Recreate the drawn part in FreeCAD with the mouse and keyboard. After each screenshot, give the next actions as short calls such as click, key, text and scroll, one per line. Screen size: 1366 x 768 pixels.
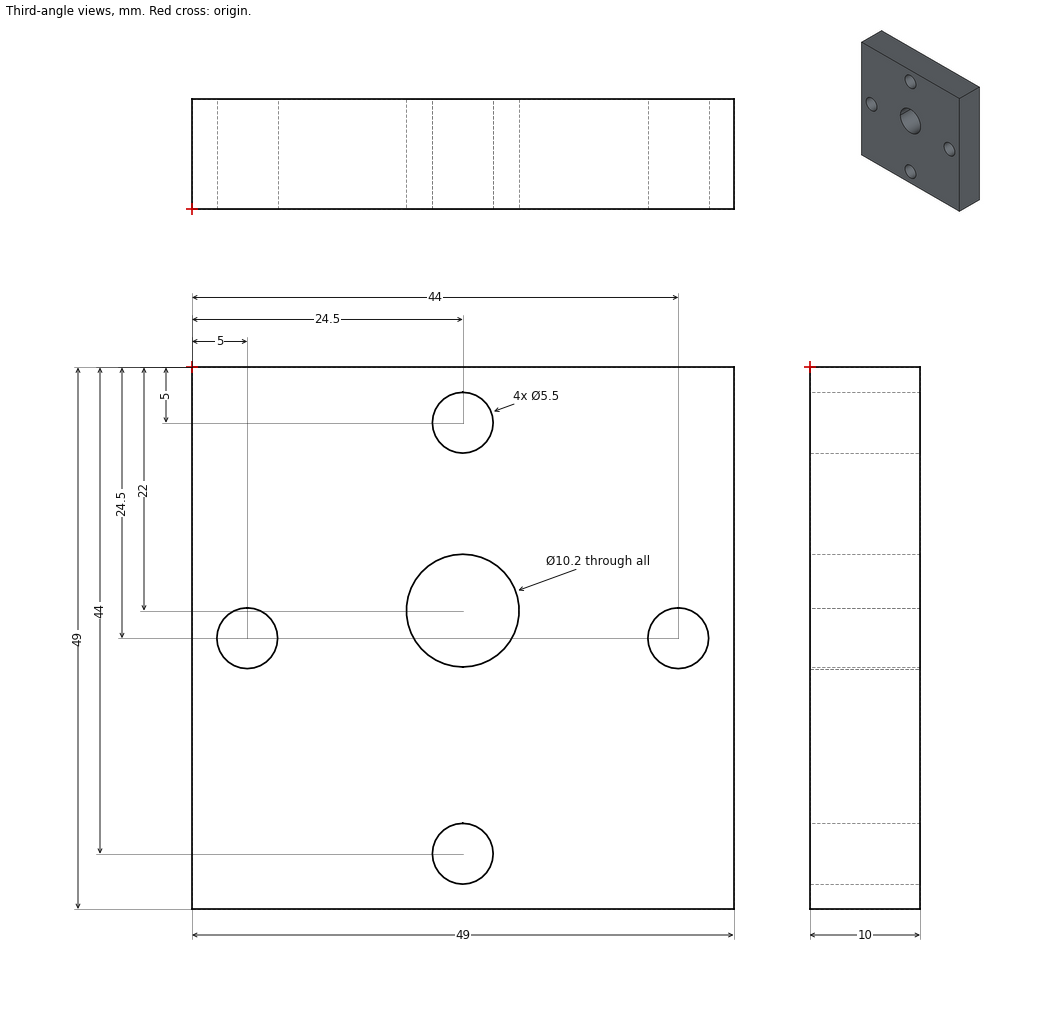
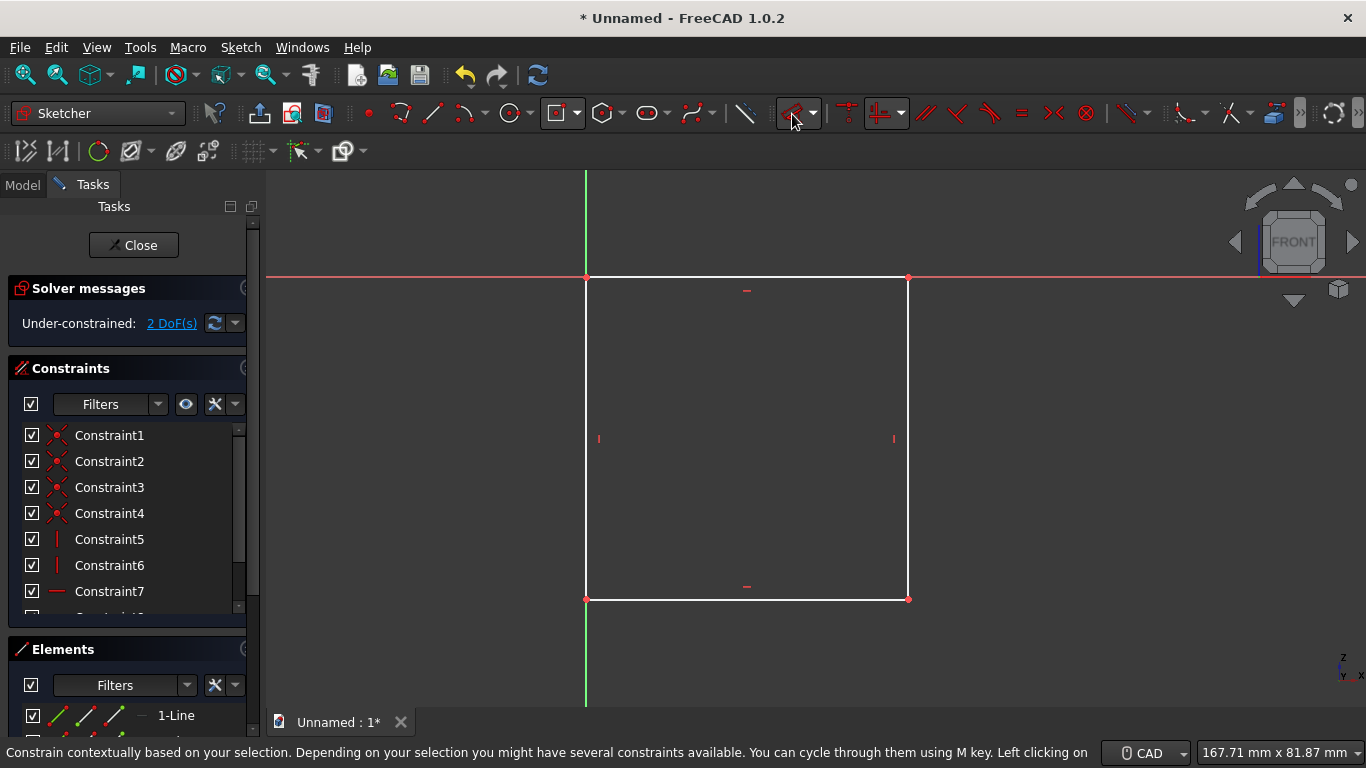
click(586, 374)
click(552, 439)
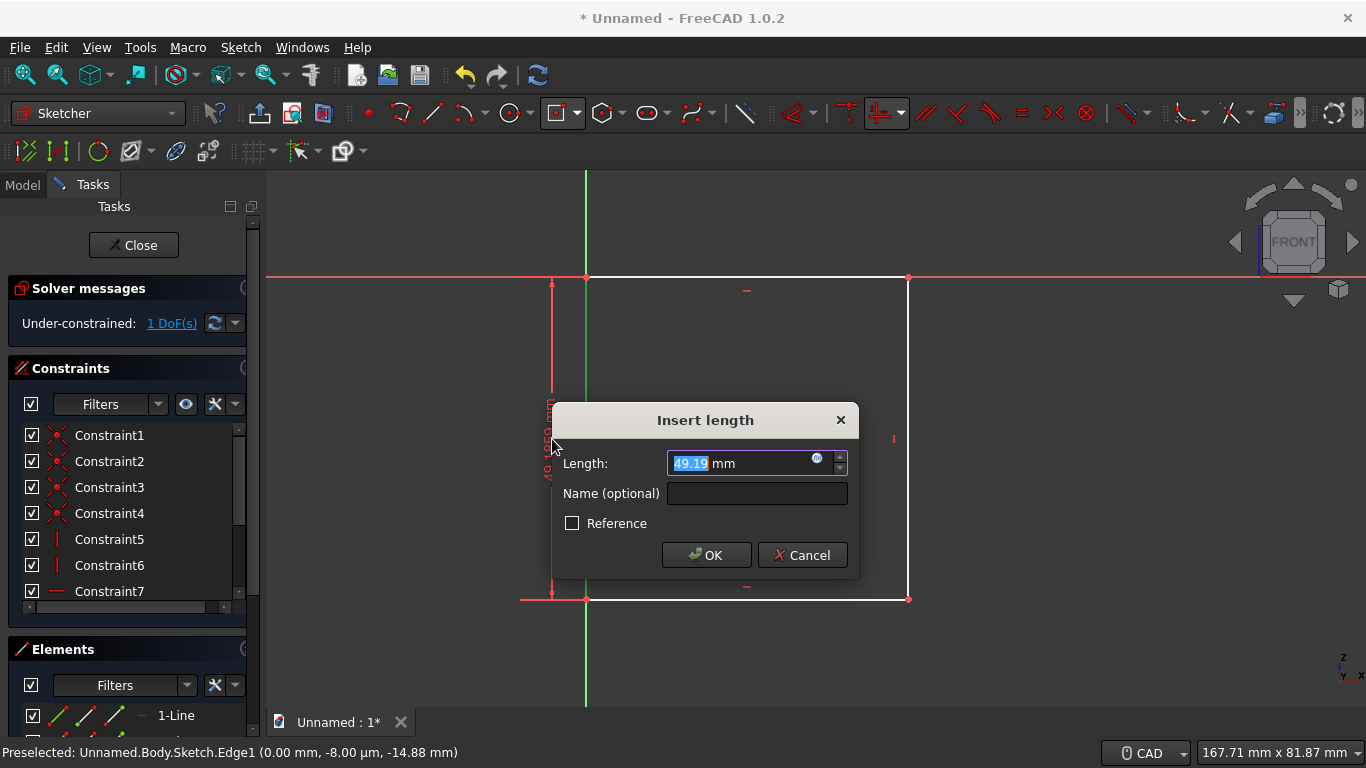
text(49)
key(Return)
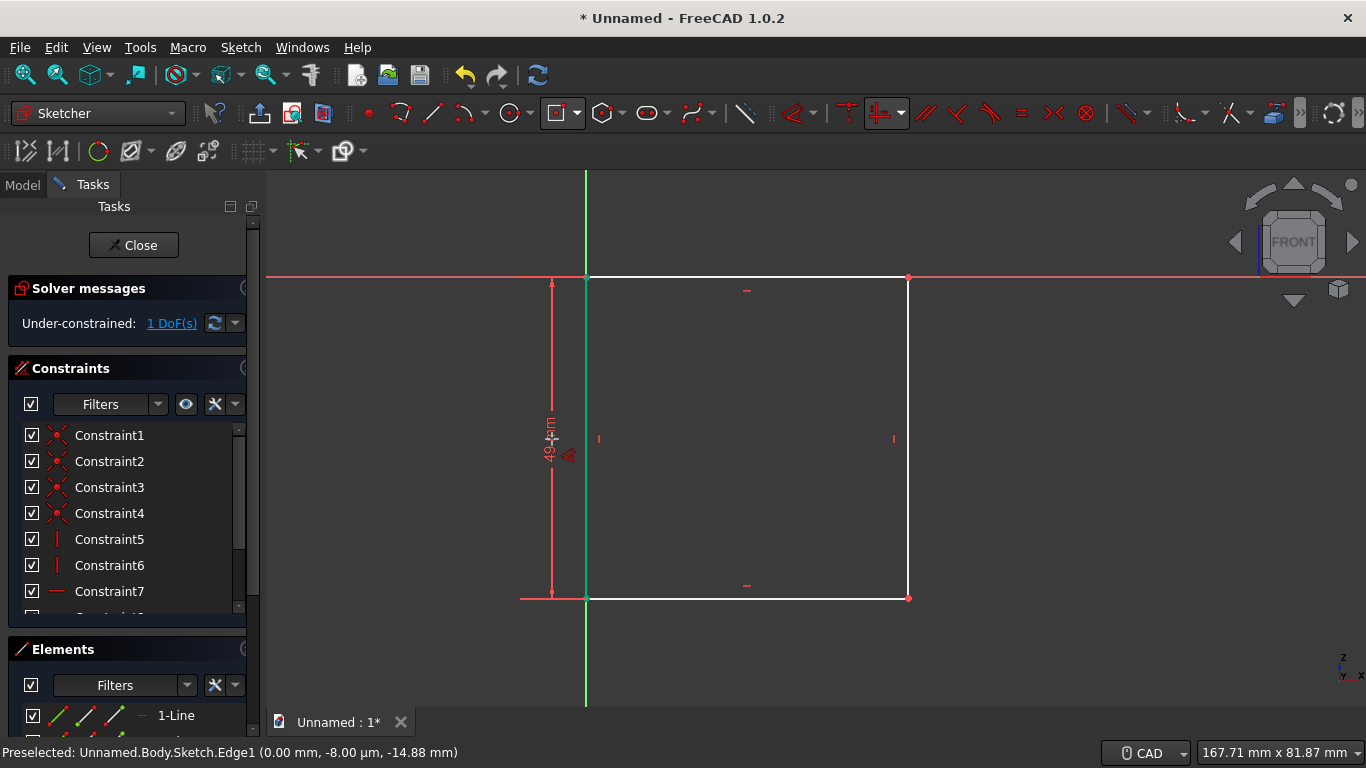
click(683, 599)
click(747, 633)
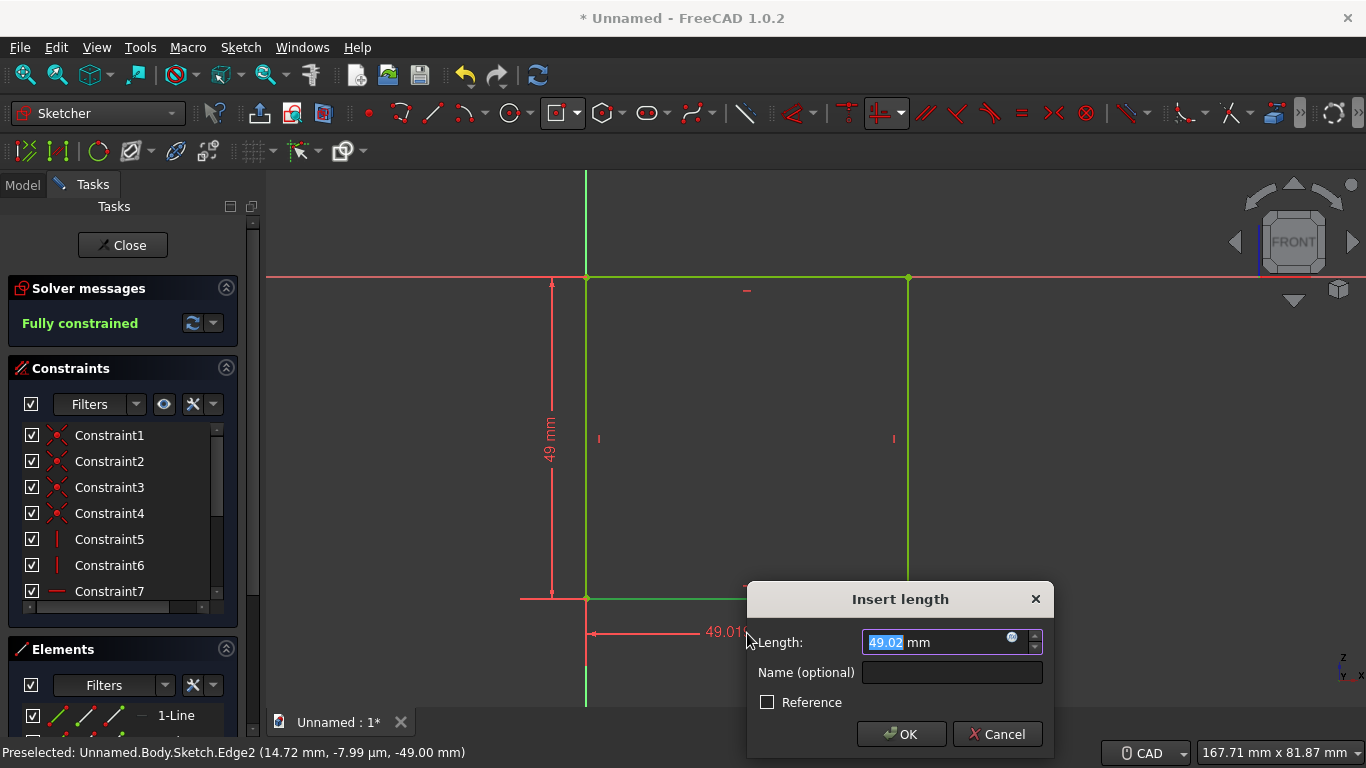
text(49)
key(Return)
key(Escape)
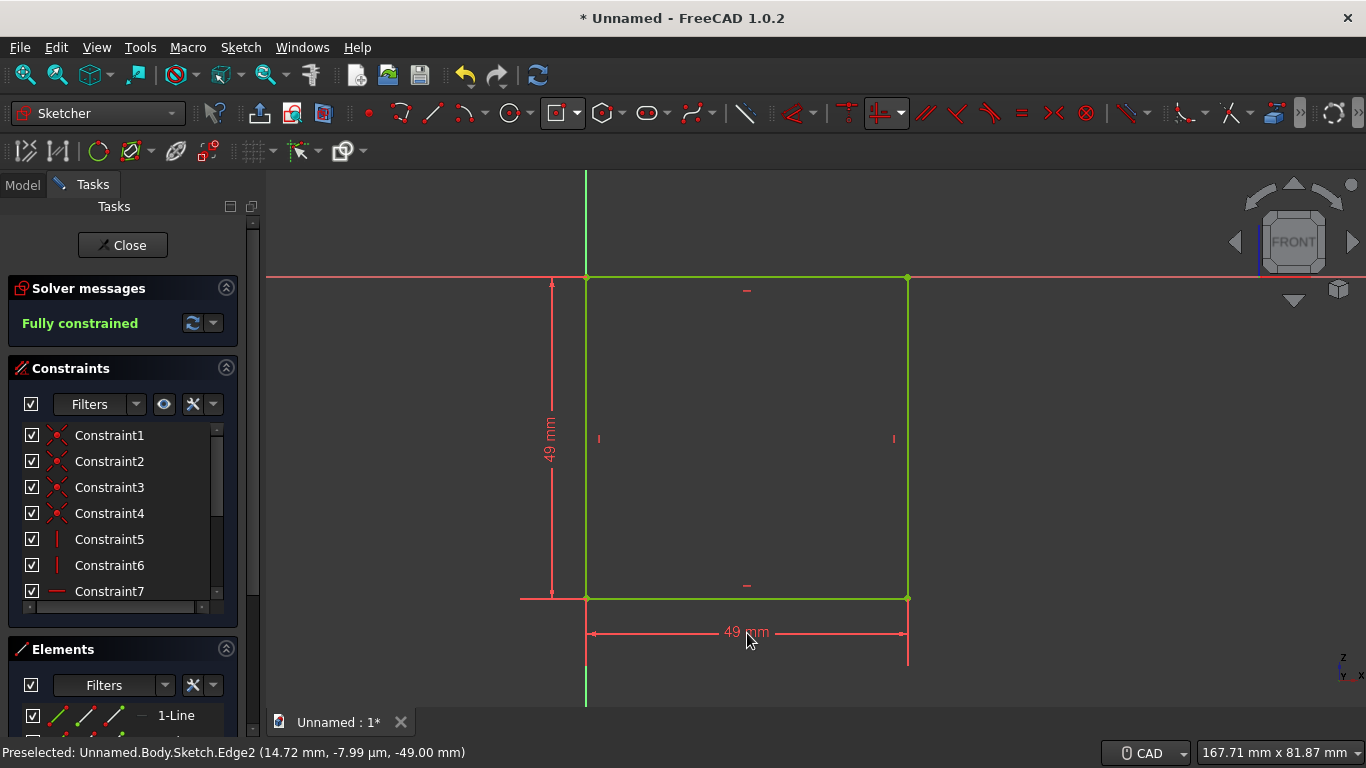
click(123, 245)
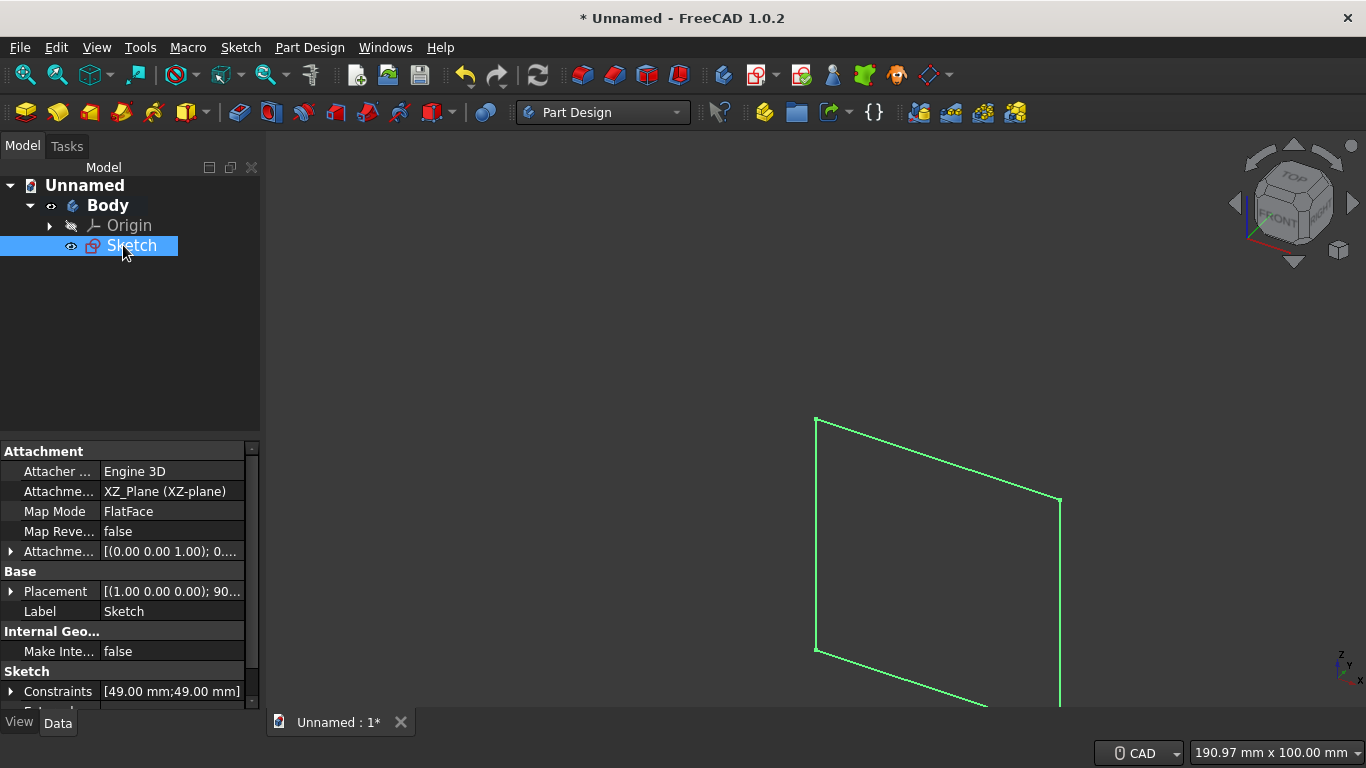
click(26, 112)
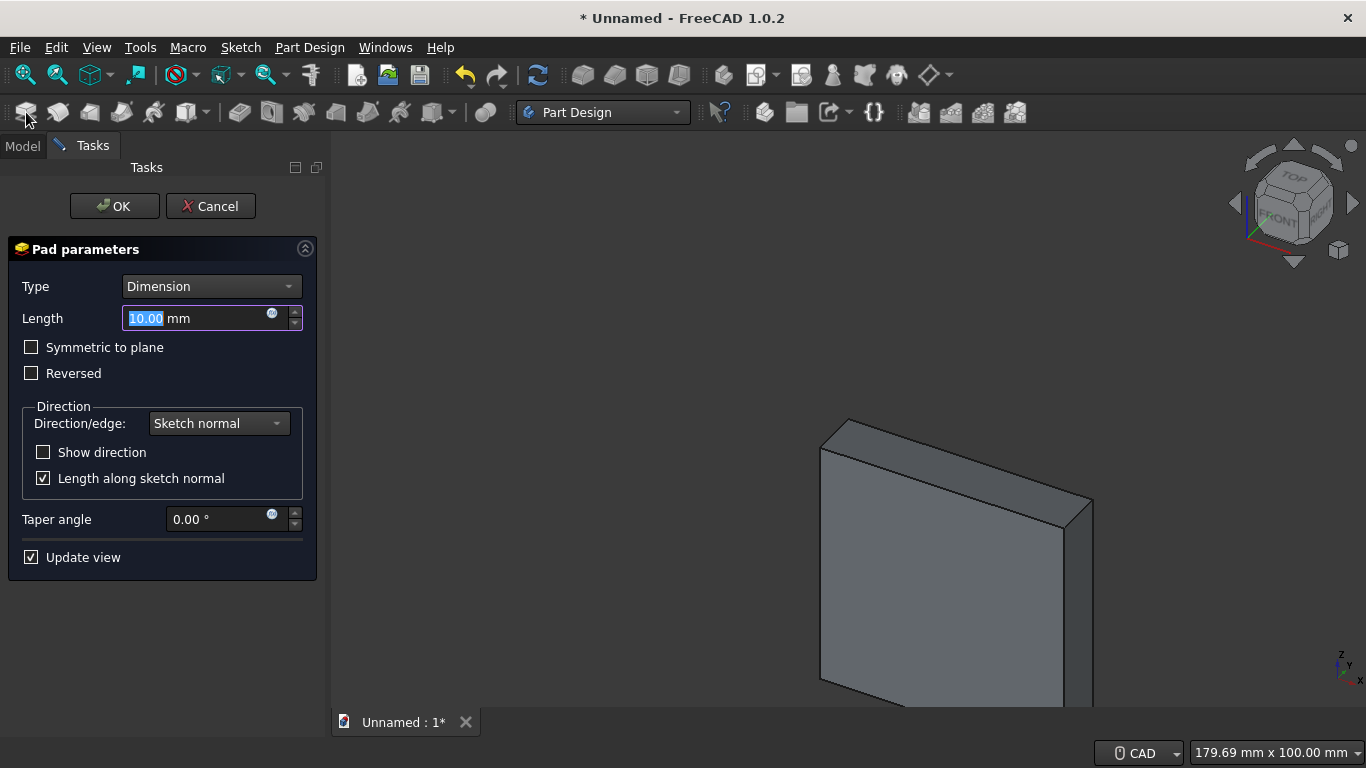
text(10)
key(Tab)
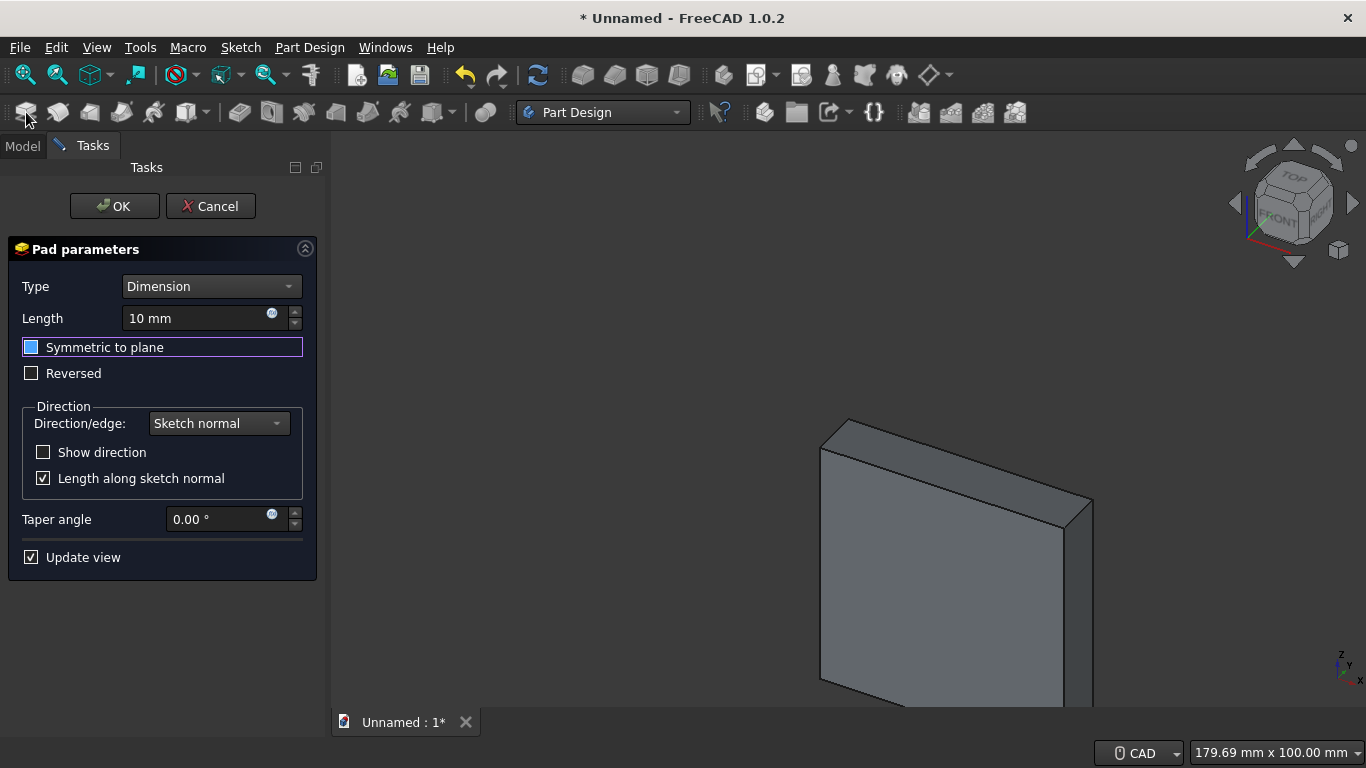
click(30, 373)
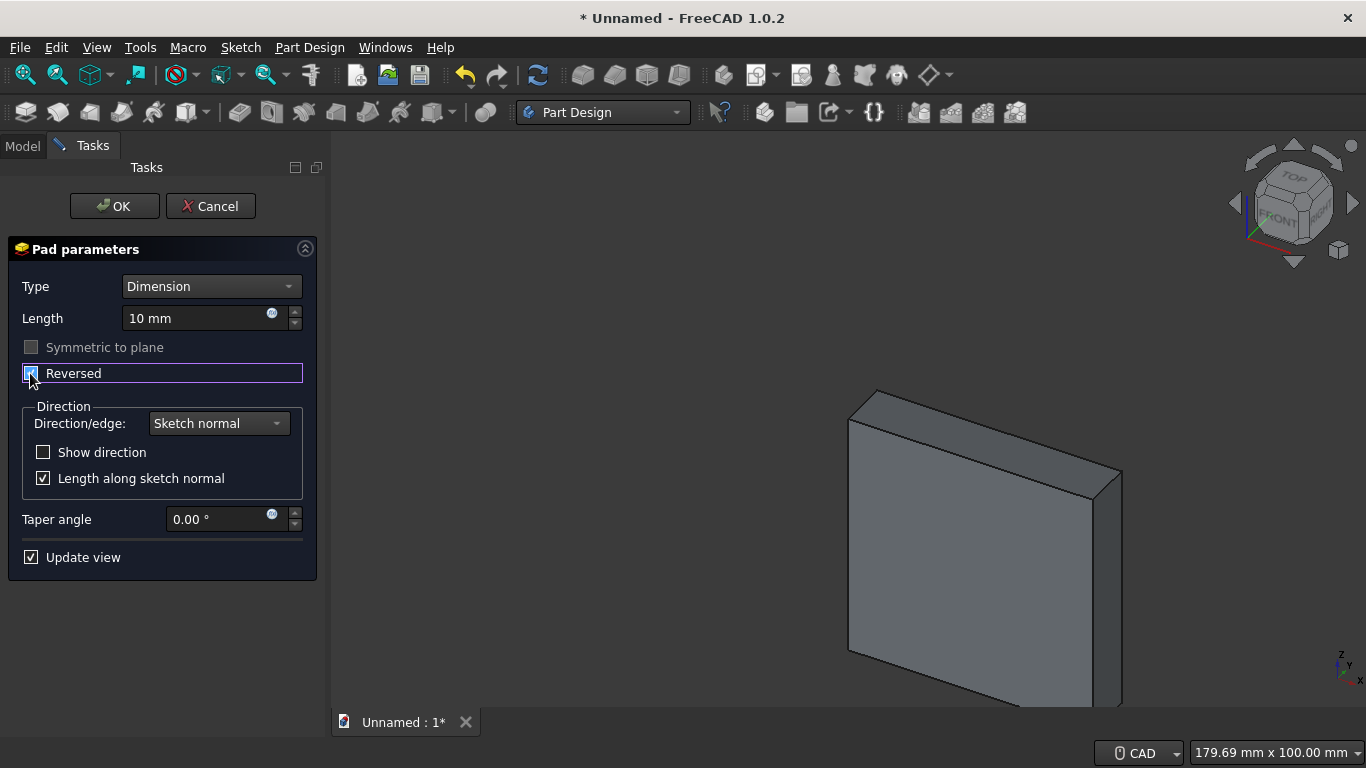
click(115, 206)